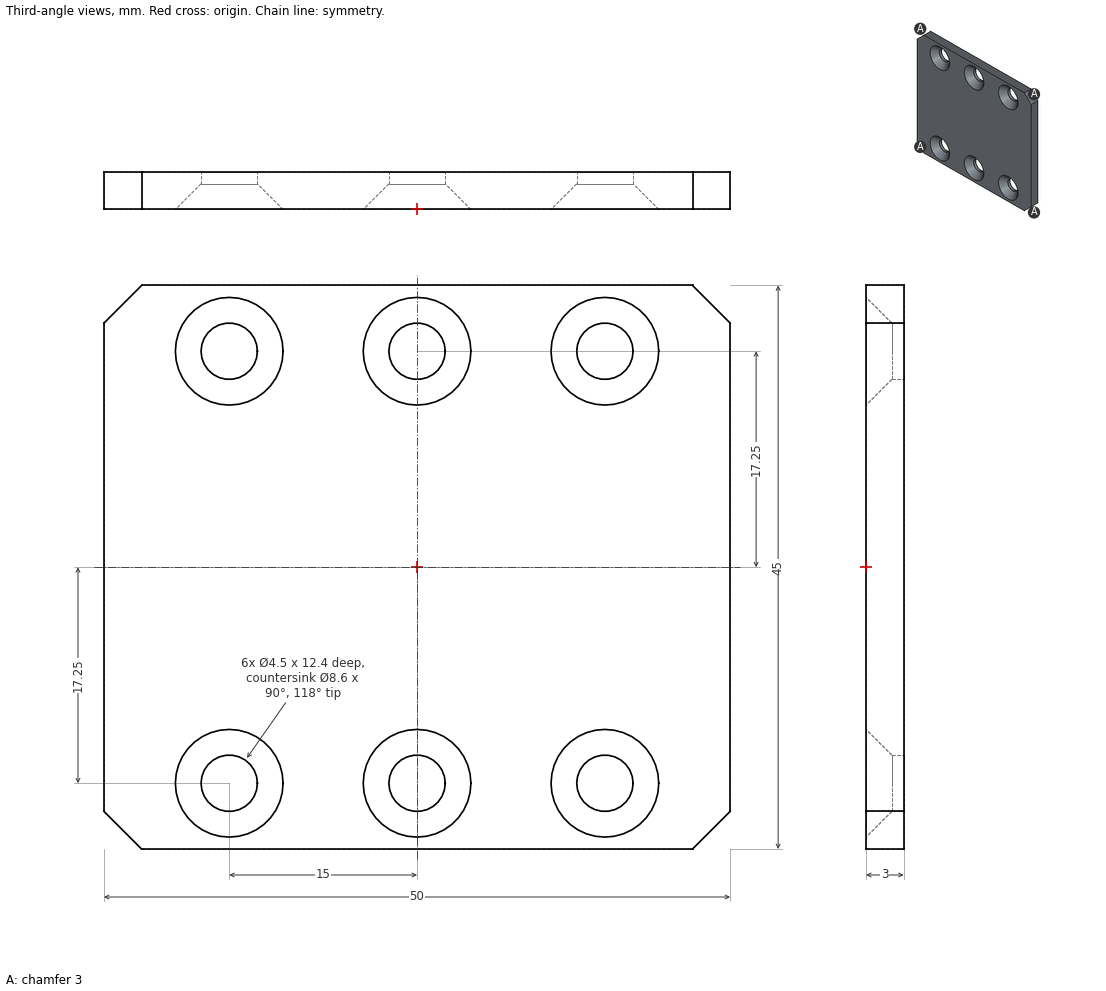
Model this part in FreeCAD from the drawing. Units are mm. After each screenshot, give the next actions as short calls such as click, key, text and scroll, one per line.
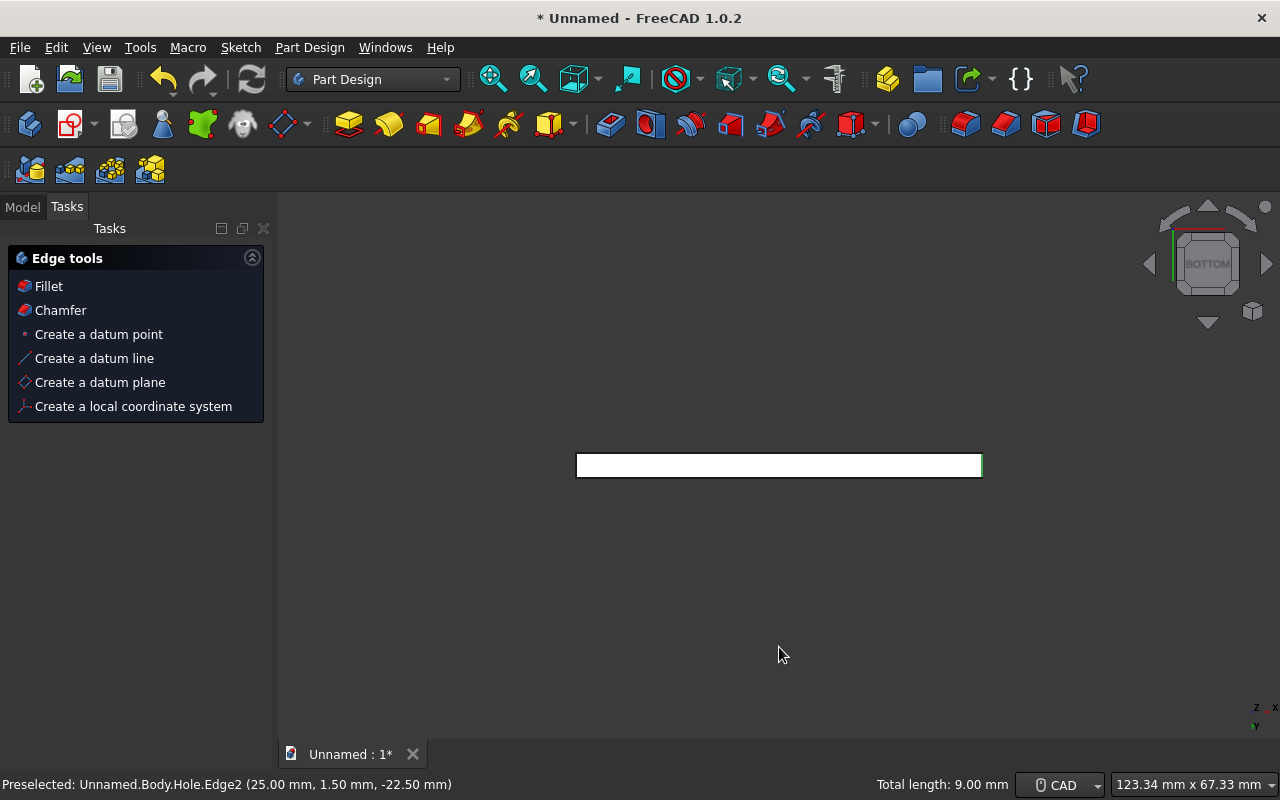
click(576, 464, ctrl)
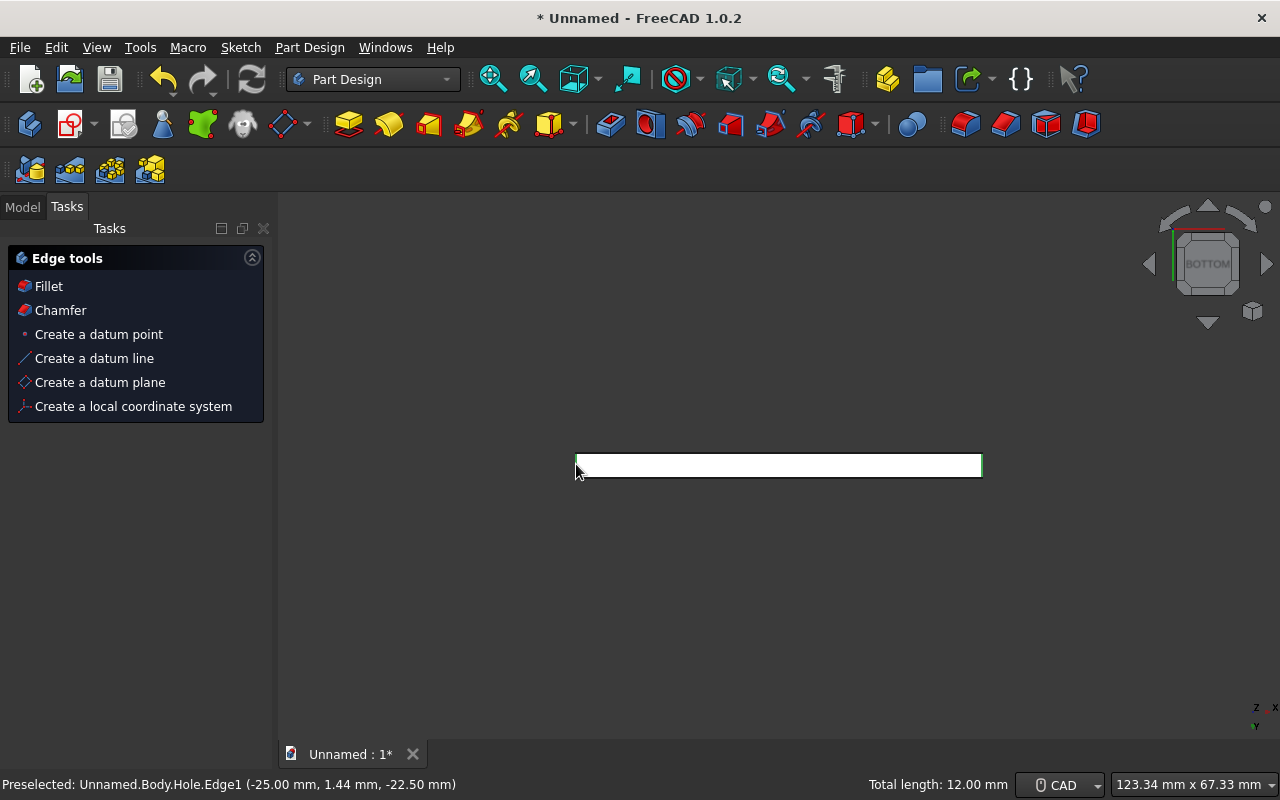
click(1006, 124)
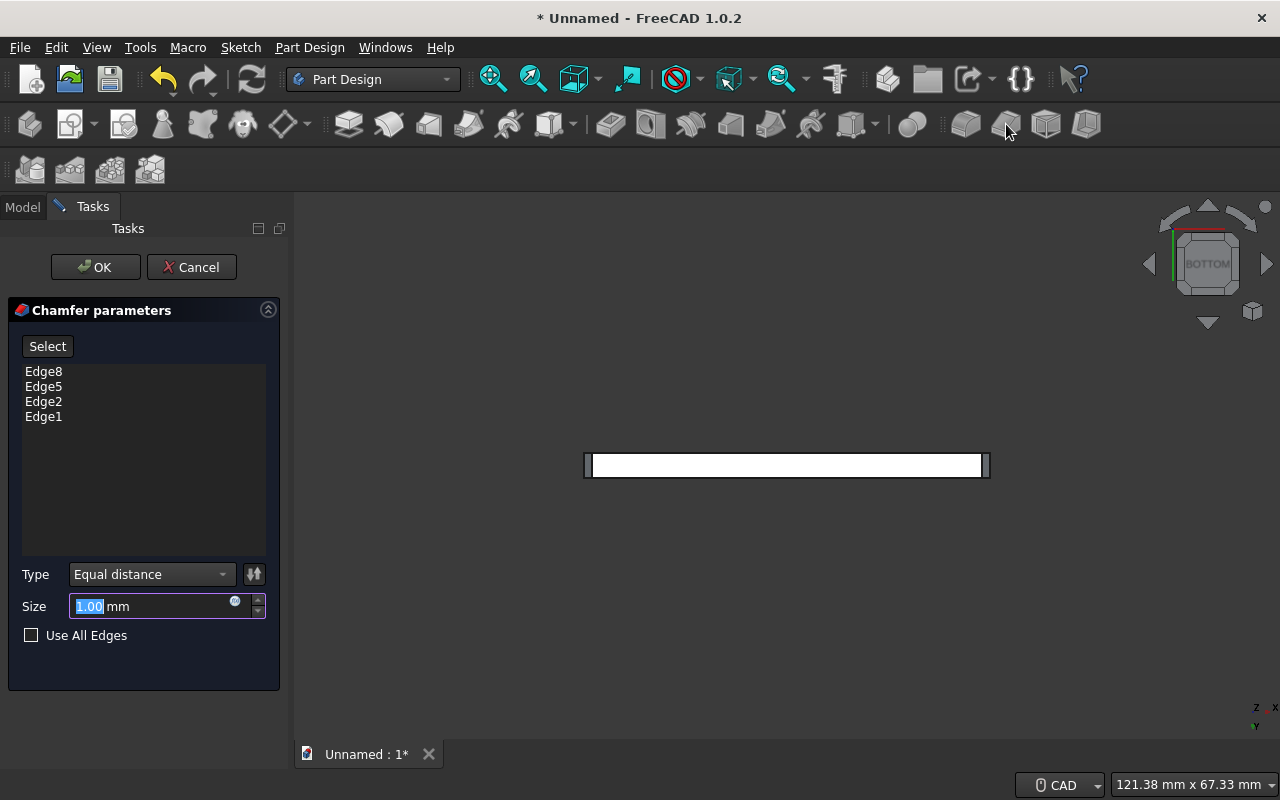
text(3)
key(Tab)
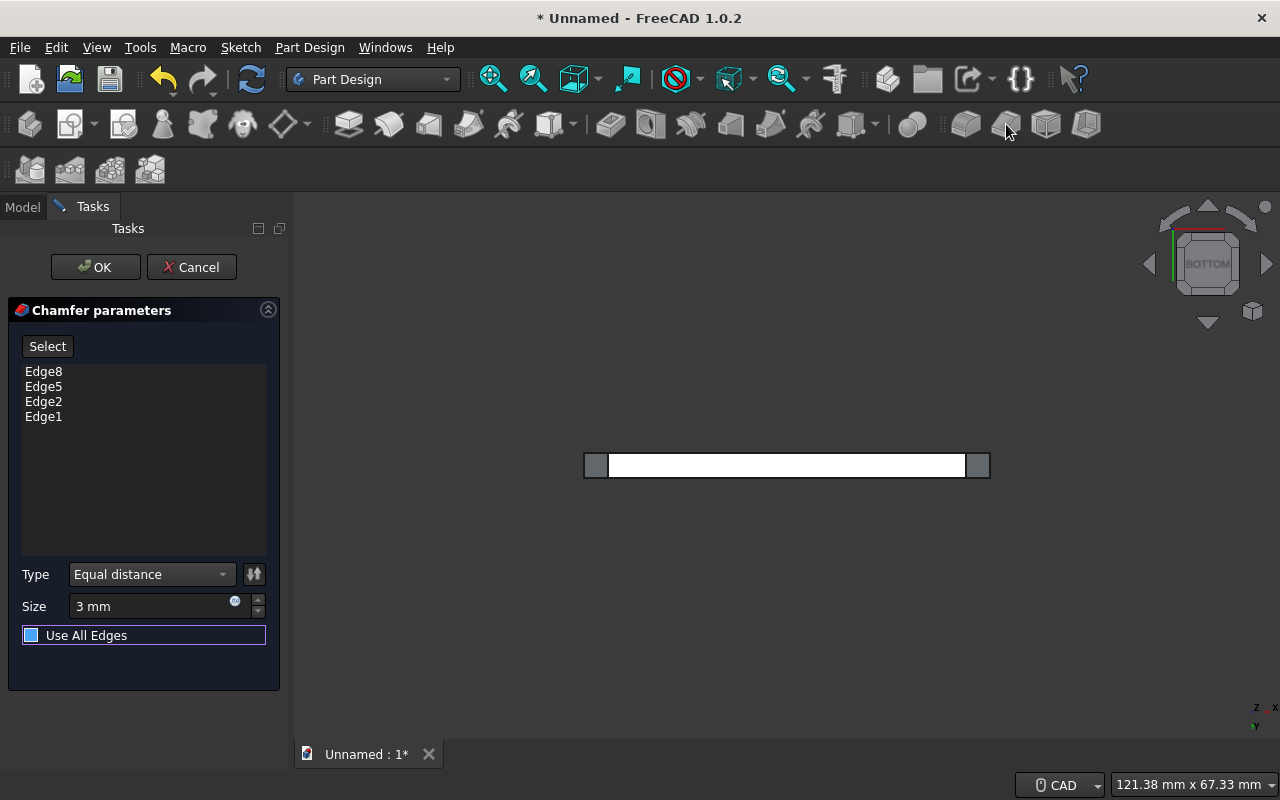
click(96, 267)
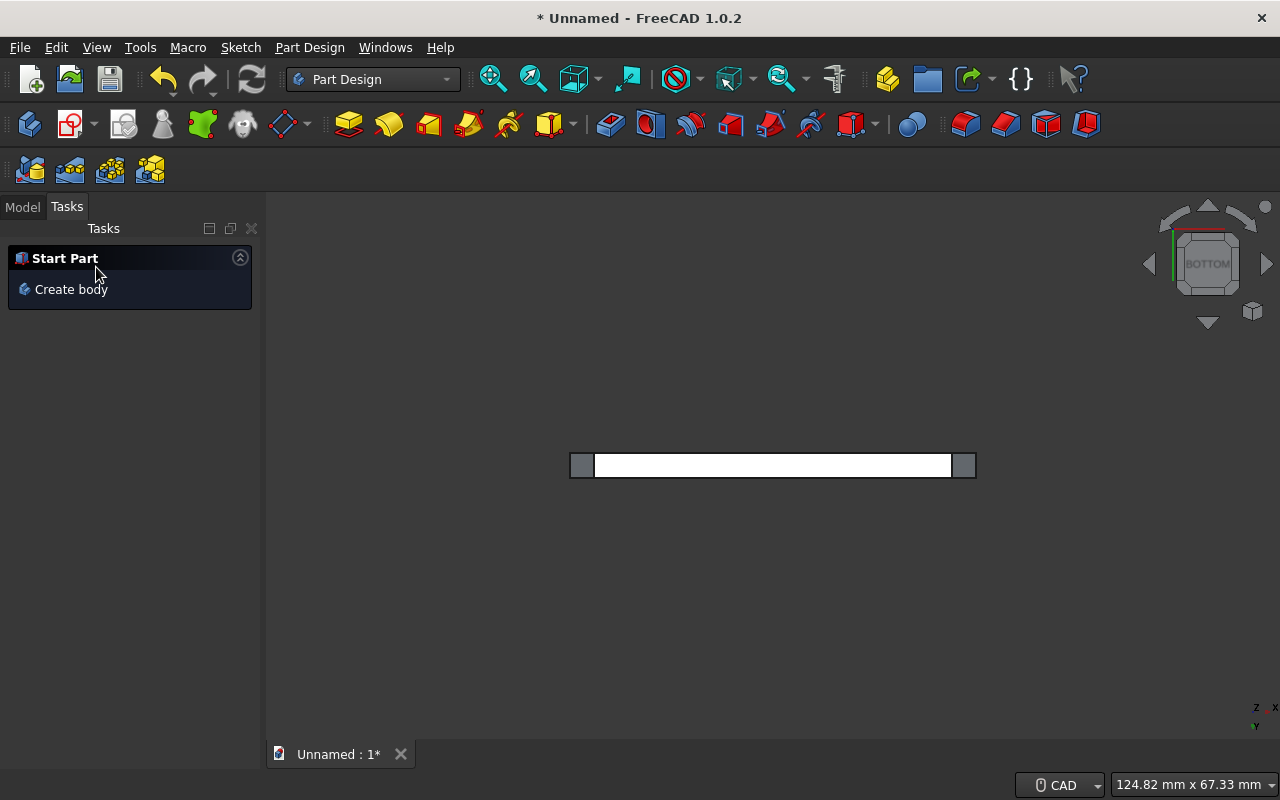
key(0)